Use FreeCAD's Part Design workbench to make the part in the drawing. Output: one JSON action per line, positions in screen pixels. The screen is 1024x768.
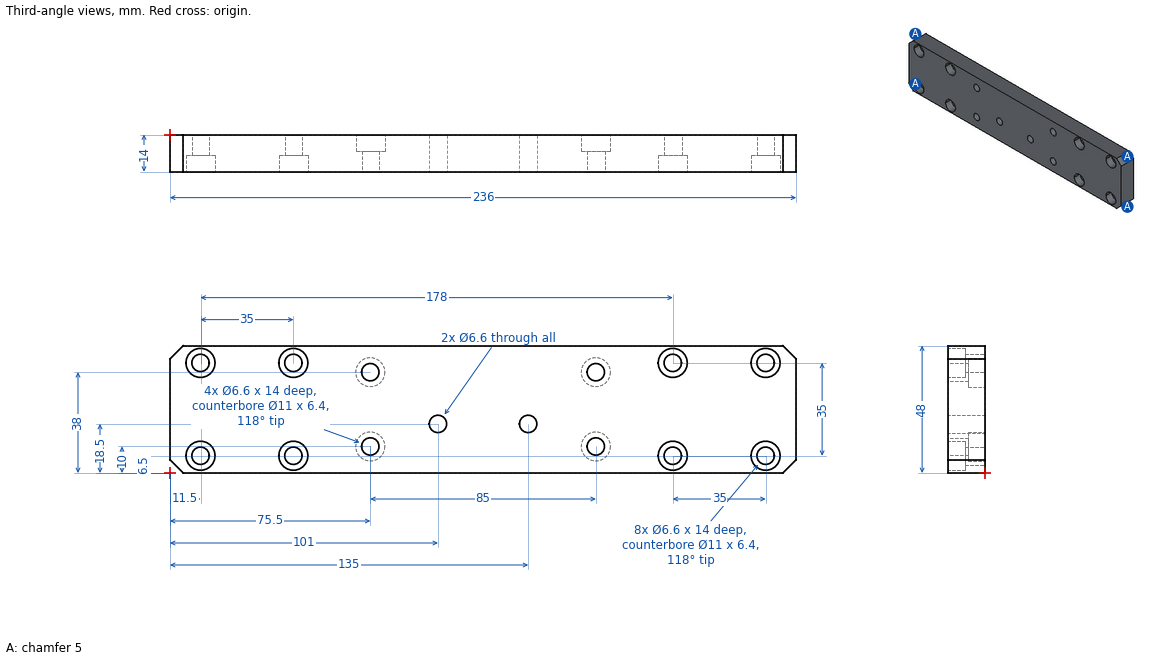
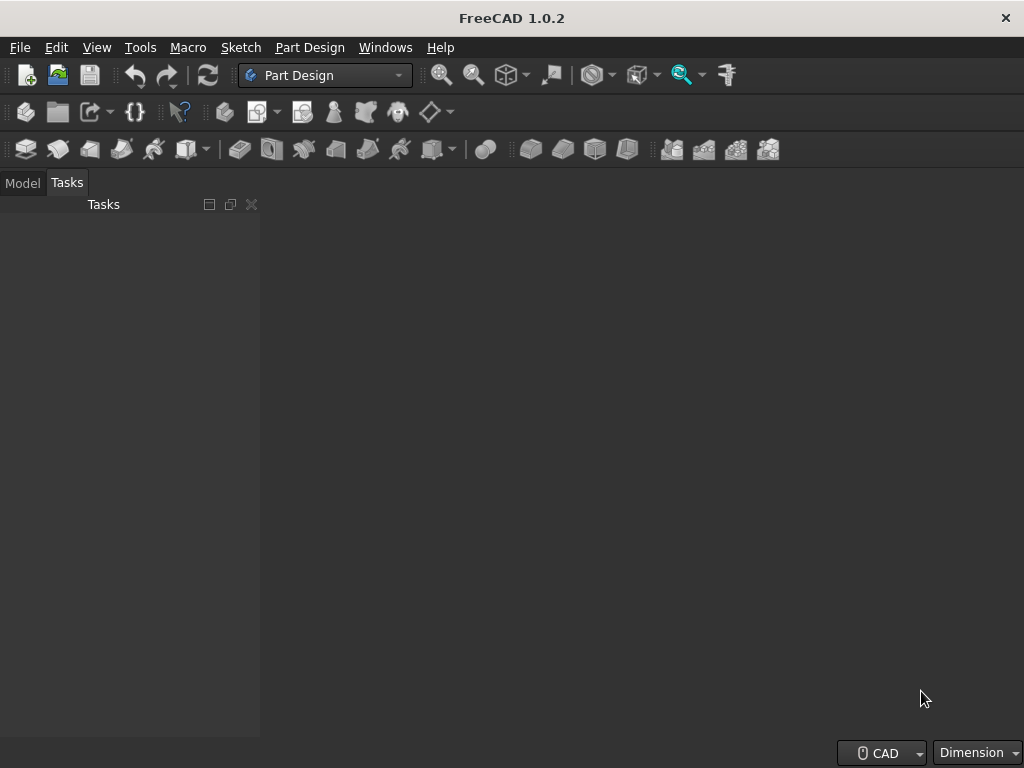
{"action": "left_click", "coordinate": [26, 76]}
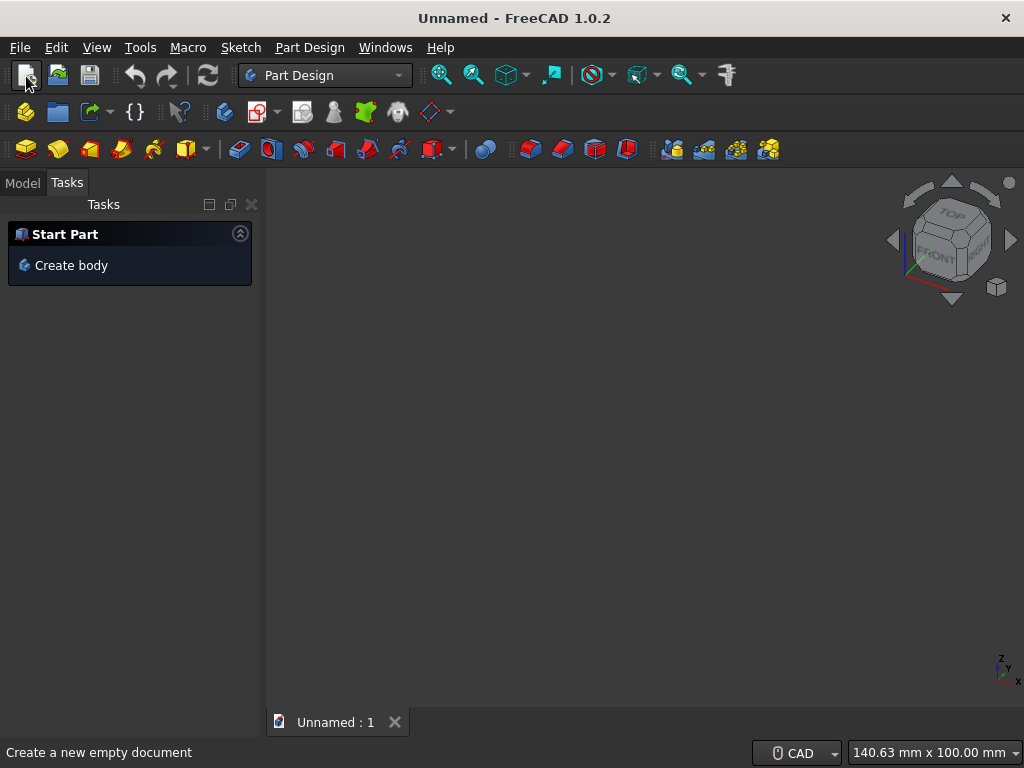
{"action": "left_click", "coordinate": [258, 112]}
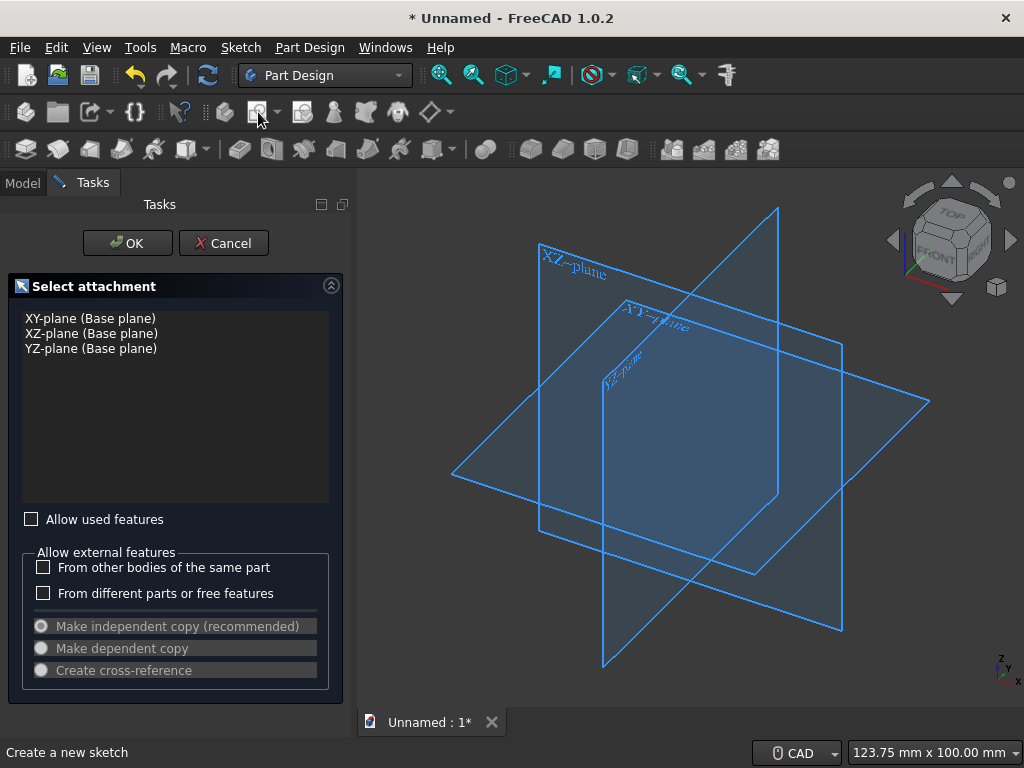
{"action": "left_click", "coordinate": [82, 318]}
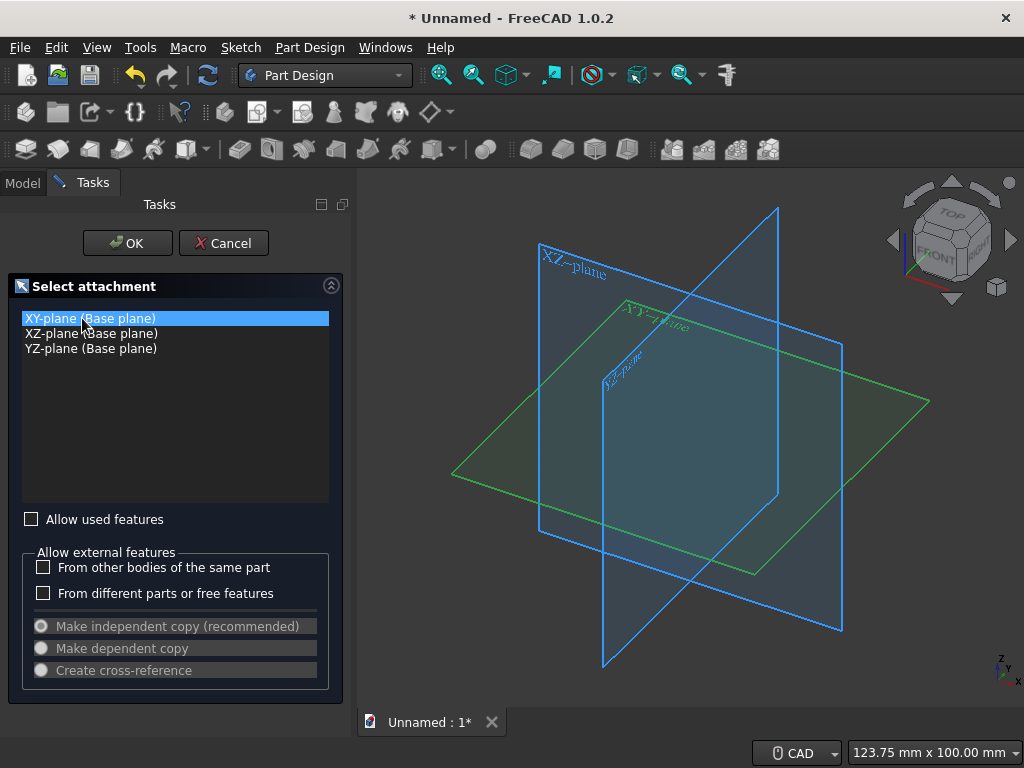
{"action": "left_click", "coordinate": [128, 243]}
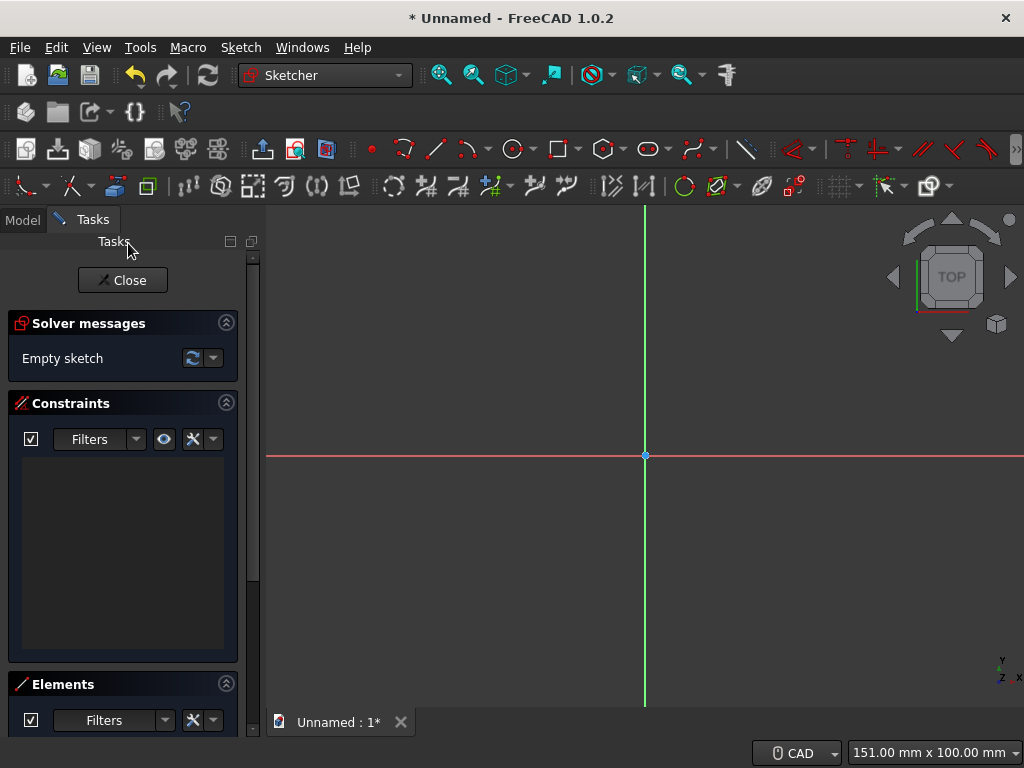
{"action": "scroll", "coordinate": [294, 441], "scroll_direction": "down", "scroll_amount": 6}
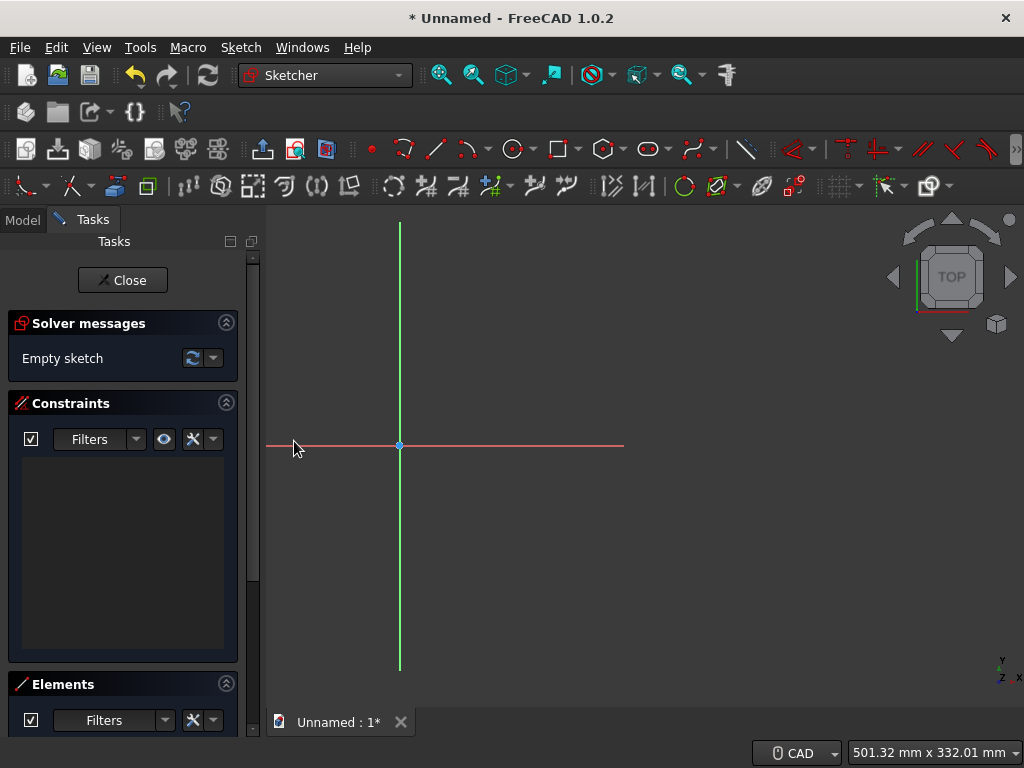
{"action": "left_click", "coordinate": [558, 150]}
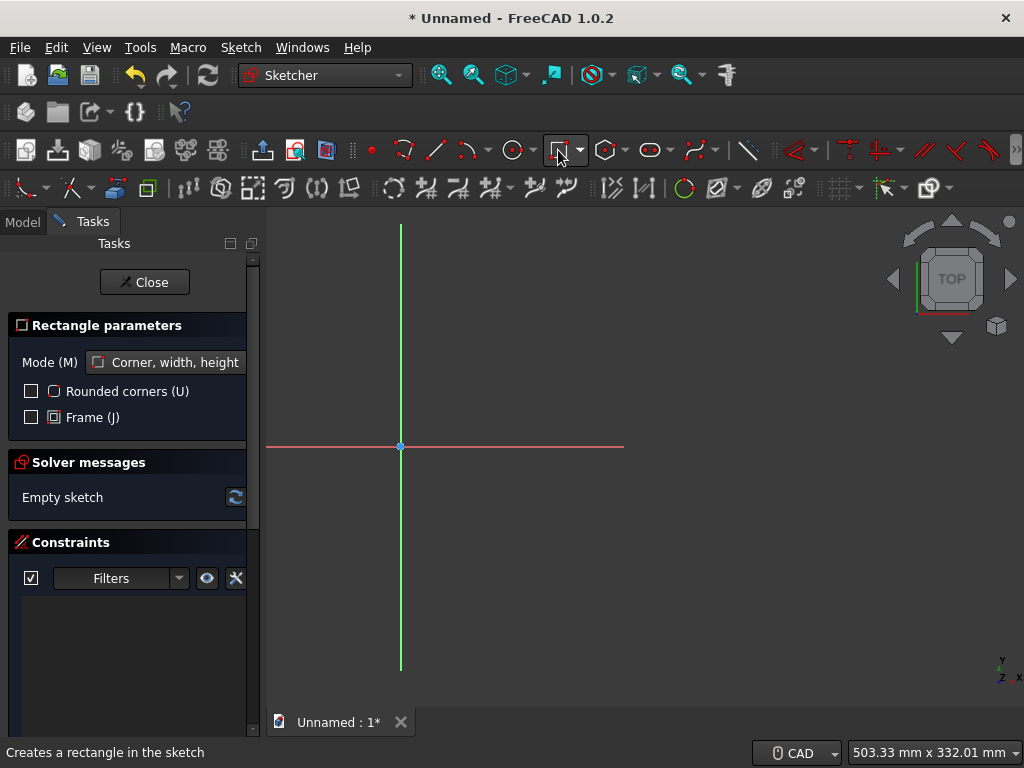
{"action": "left_click", "coordinate": [401, 447]}
{"action": "left_click", "coordinate": [756, 468]}
{"action": "key", "text": "Escape"}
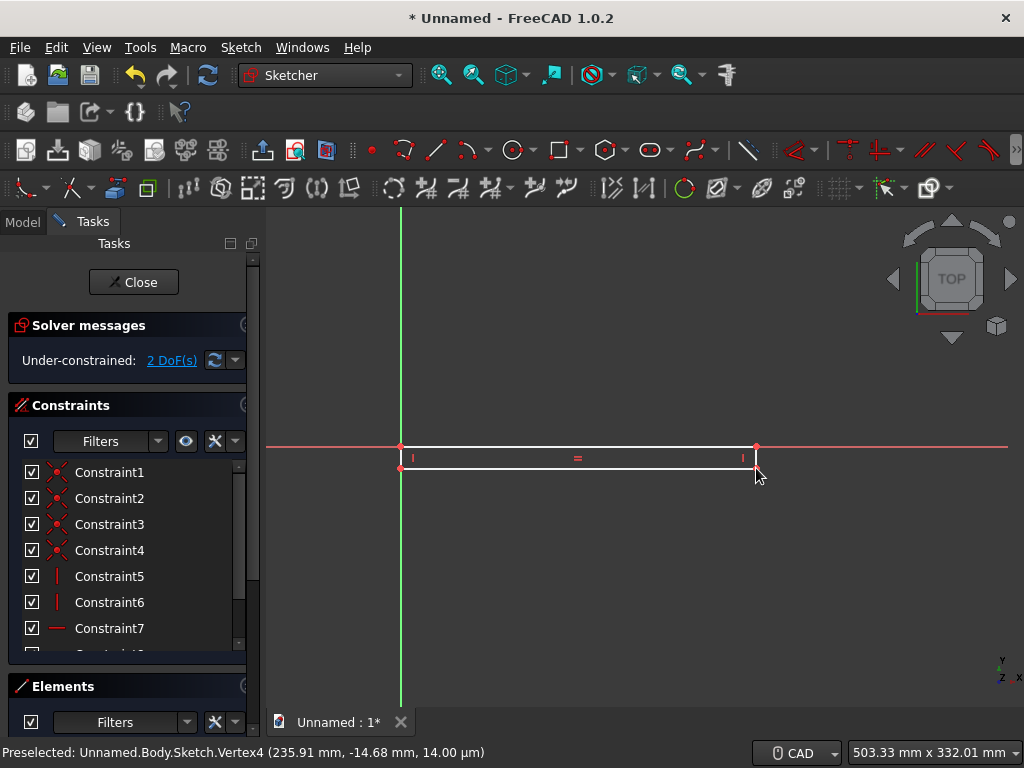
{"action": "left_click", "coordinate": [794, 150]}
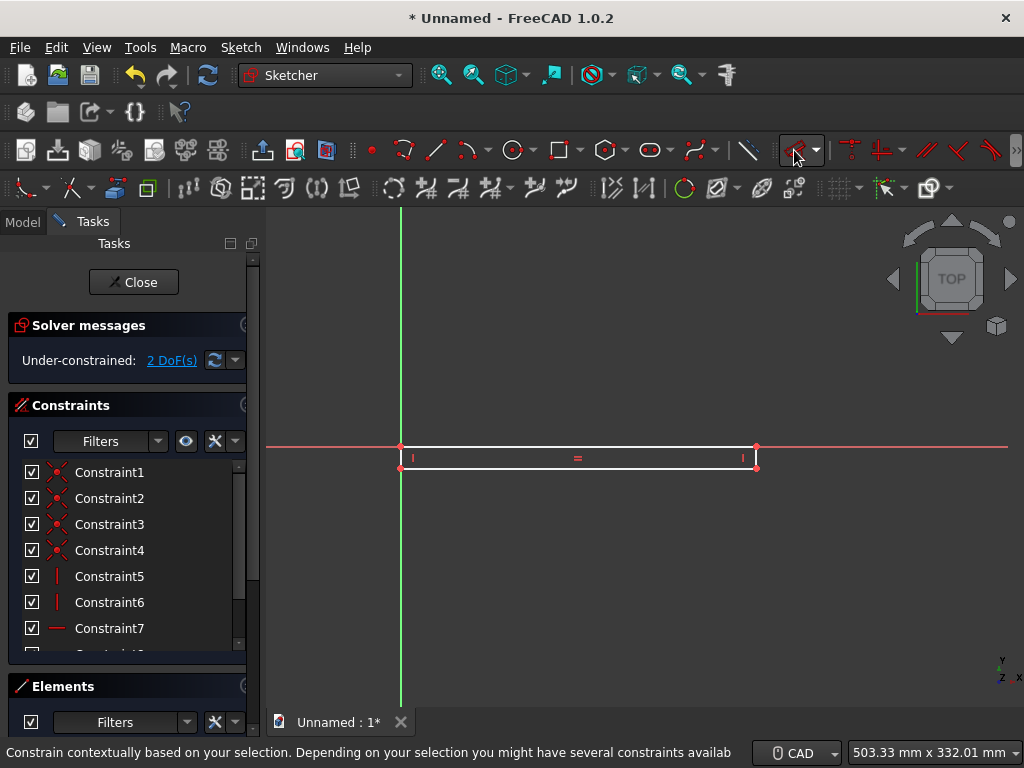
{"action": "scroll", "coordinate": [401, 458], "scroll_direction": "up", "scroll_amount": 4}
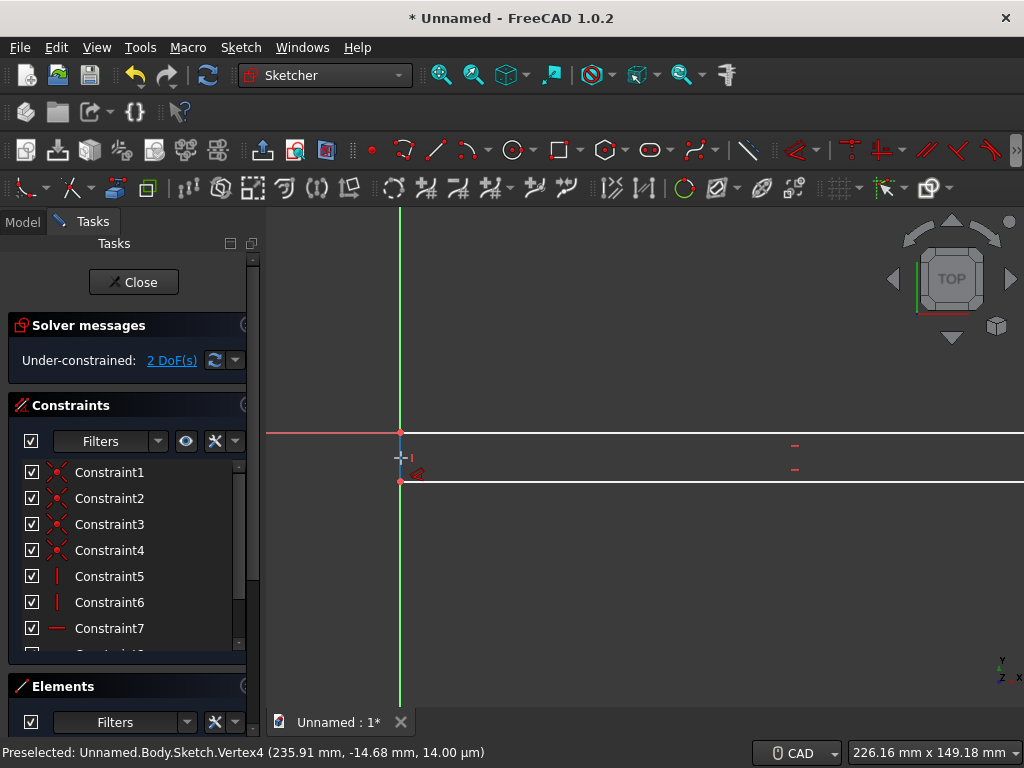
{"action": "left_click", "coordinate": [400, 457]}
{"action": "left_click", "coordinate": [366, 457]}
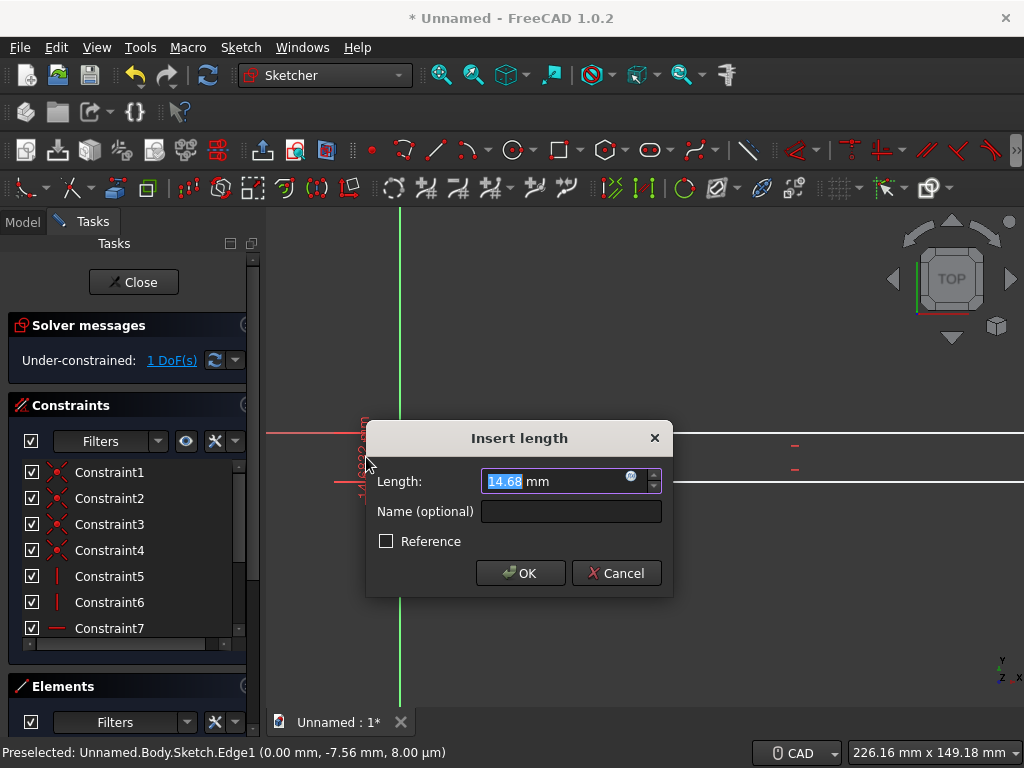
{"action": "type", "text": "14"}
{"action": "key", "text": "Return"}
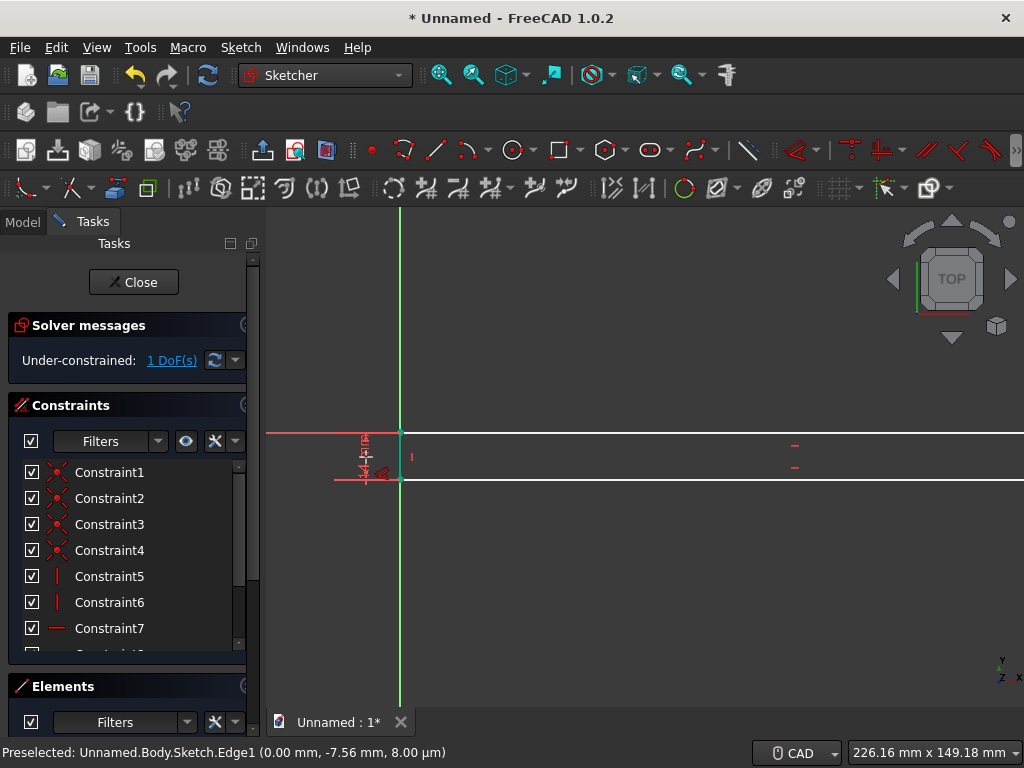
{"action": "left_click", "coordinate": [637, 480]}
{"action": "left_click", "coordinate": [630, 514]}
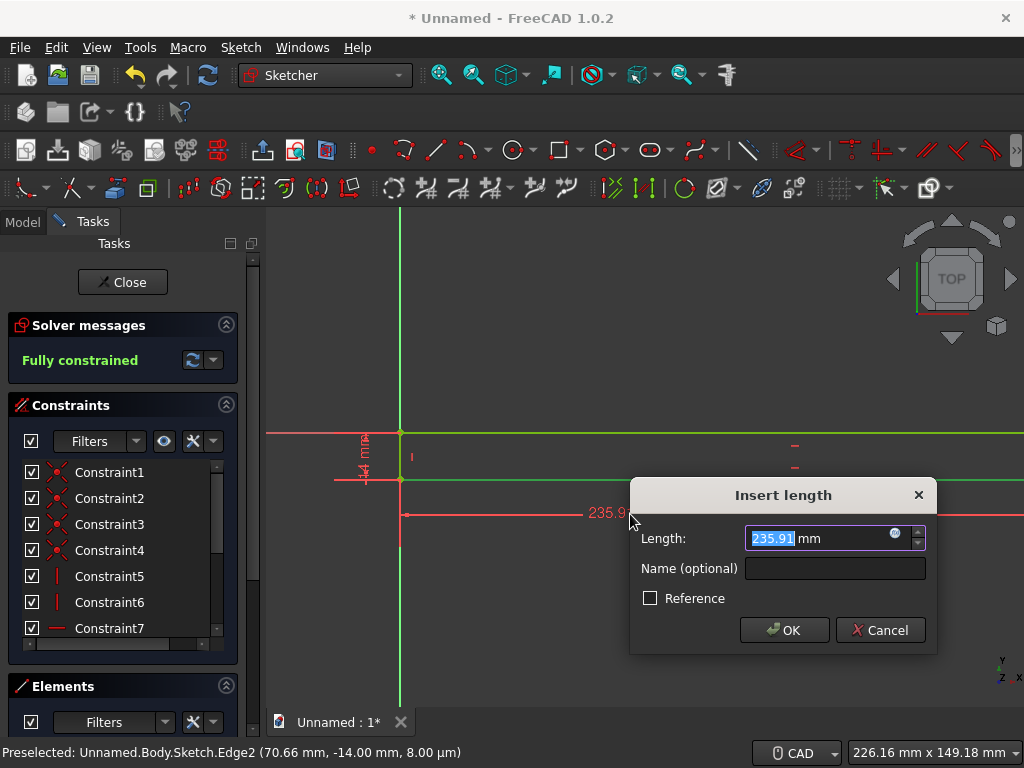
{"action": "type", "text": "236"}
{"action": "key", "text": "Return"}
{"action": "key", "text": "Escape"}